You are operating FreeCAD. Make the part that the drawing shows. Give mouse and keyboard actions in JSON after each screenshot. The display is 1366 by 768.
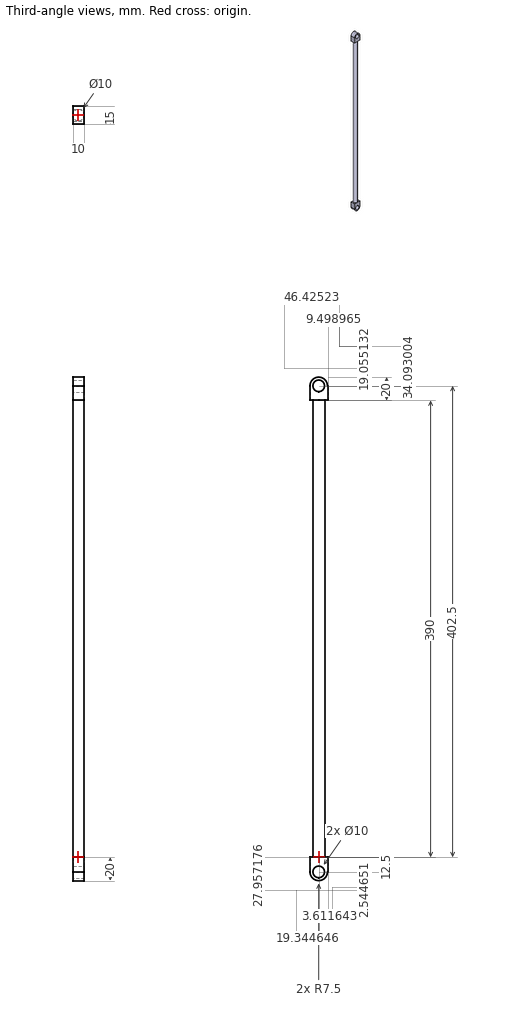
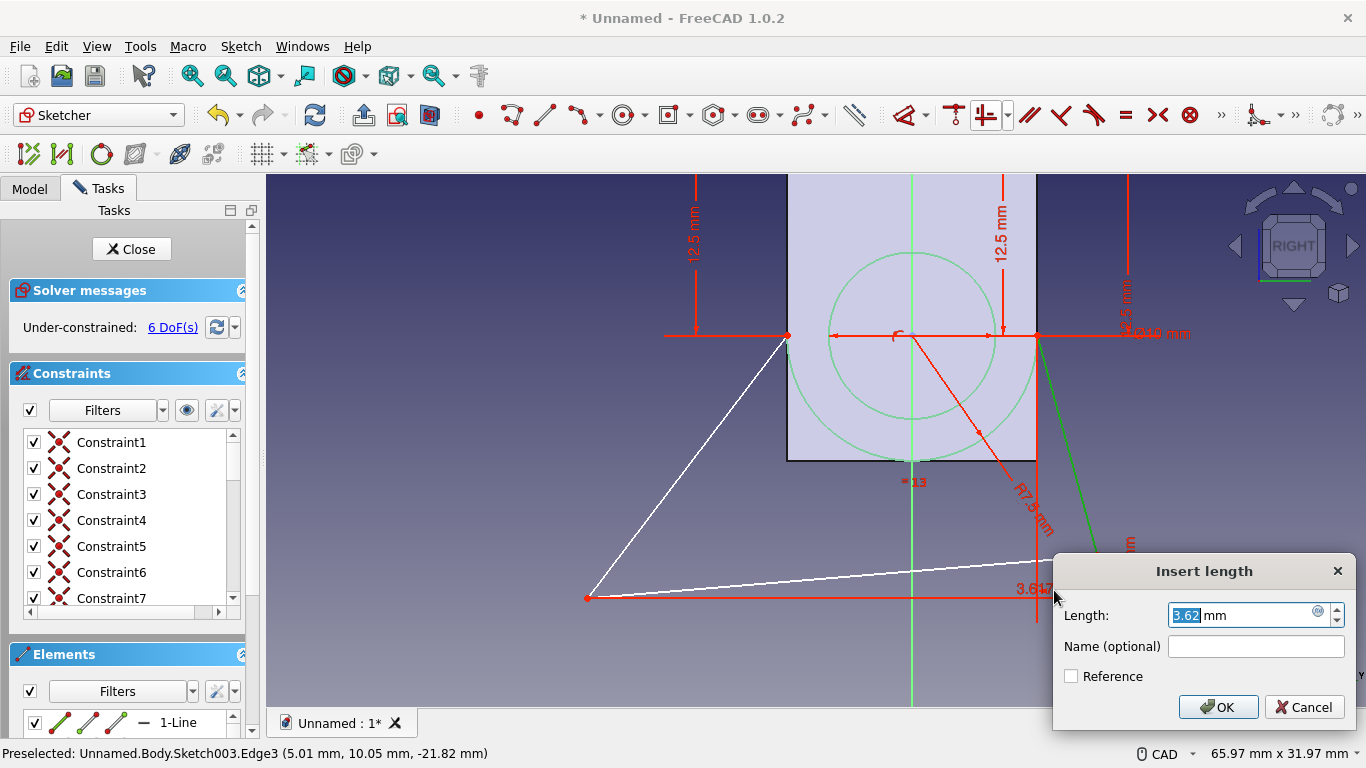
{"action": "type", "text": "3.611643"}
{"action": "key", "text": "Return"}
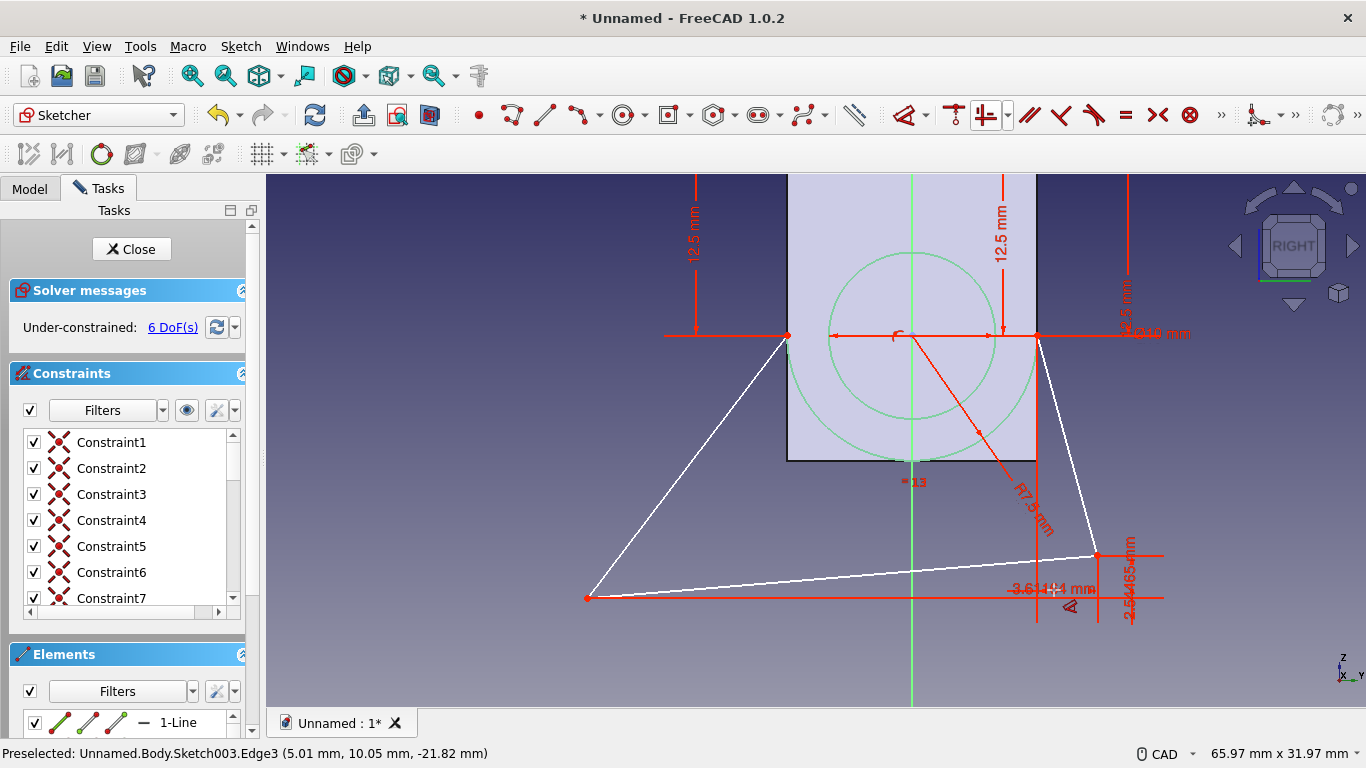
{"action": "scroll", "coordinate": [744, 635], "scroll_direction": "down", "scroll_amount": 15}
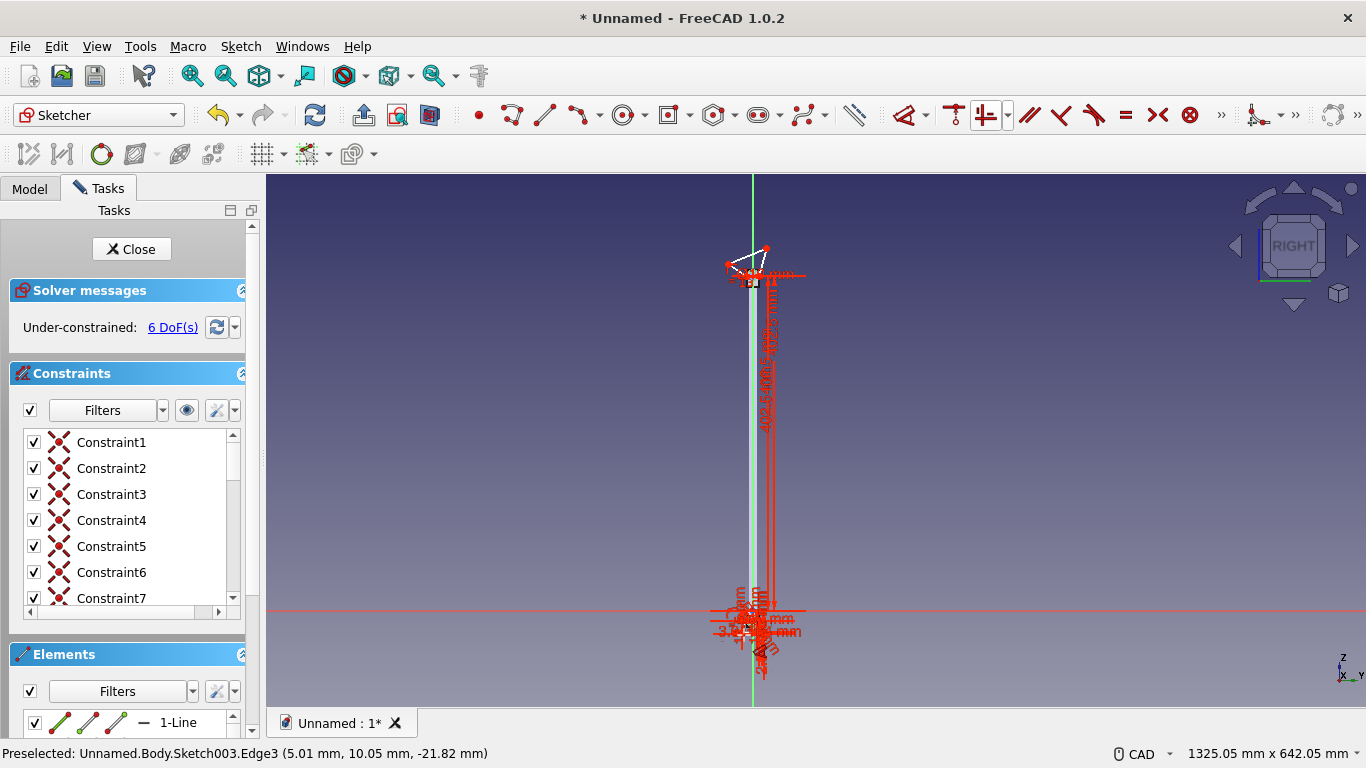
{"action": "scroll", "coordinate": [761, 268], "scroll_direction": "up", "scroll_amount": 9}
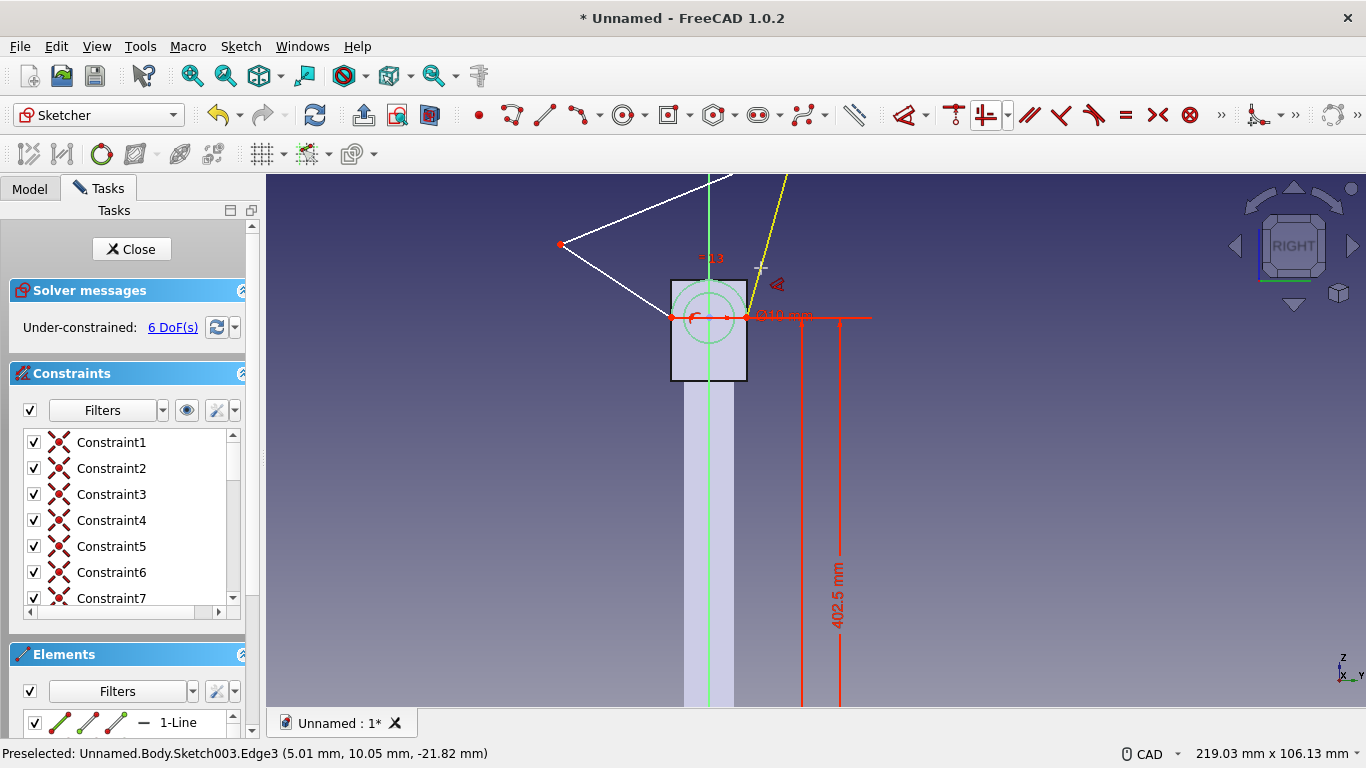
{"action": "left_click", "coordinate": [761, 267]}
{"action": "left_click", "coordinate": [770, 352]}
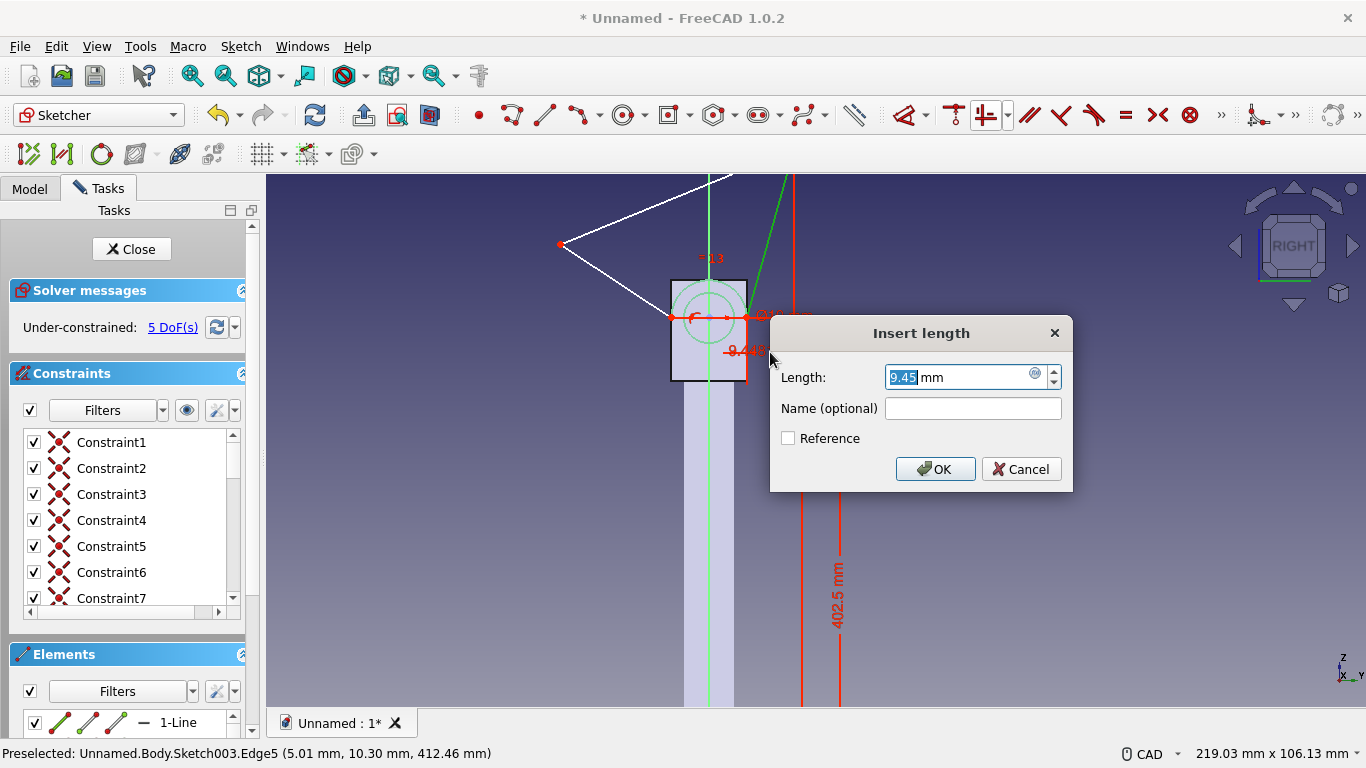
{"action": "type", "text": "9.498965"}
{"action": "key", "text": "Return"}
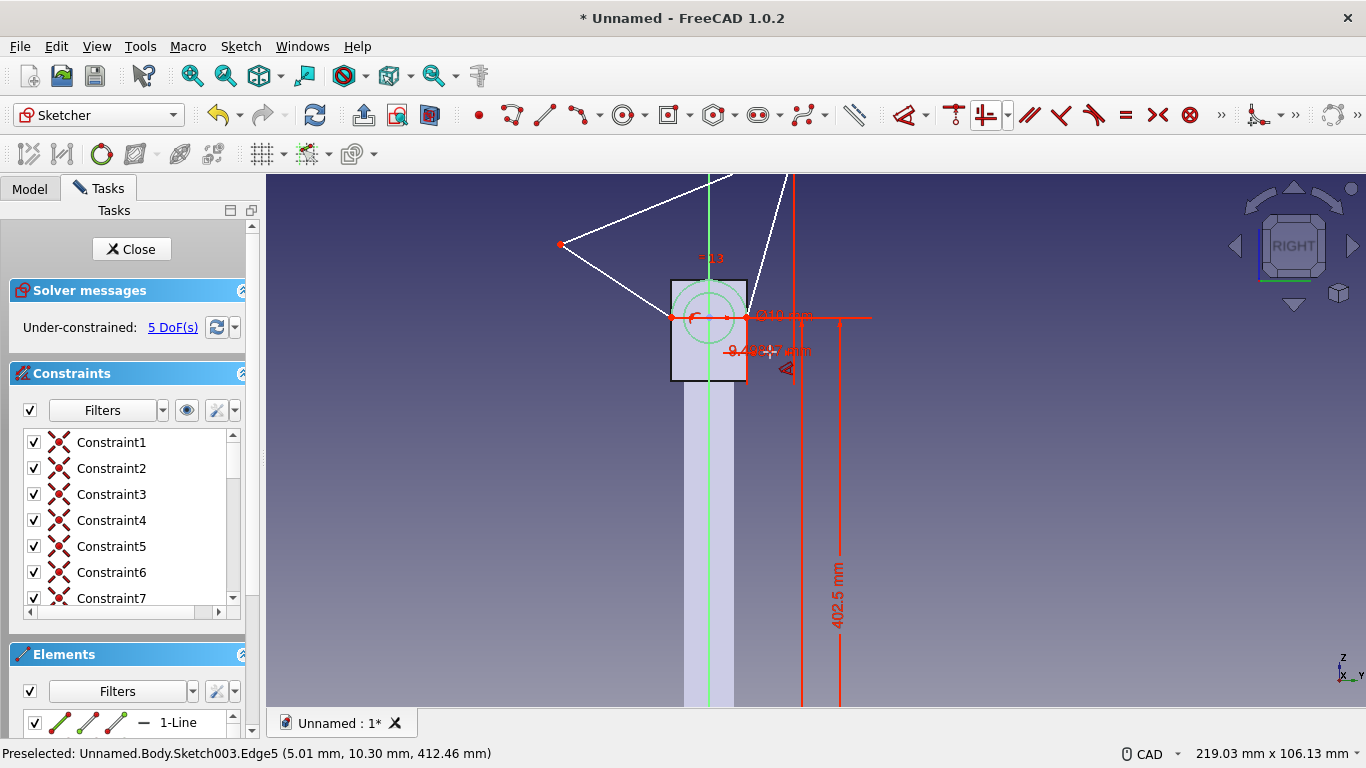
{"action": "scroll", "coordinate": [758, 304], "scroll_direction": "down", "scroll_amount": 10}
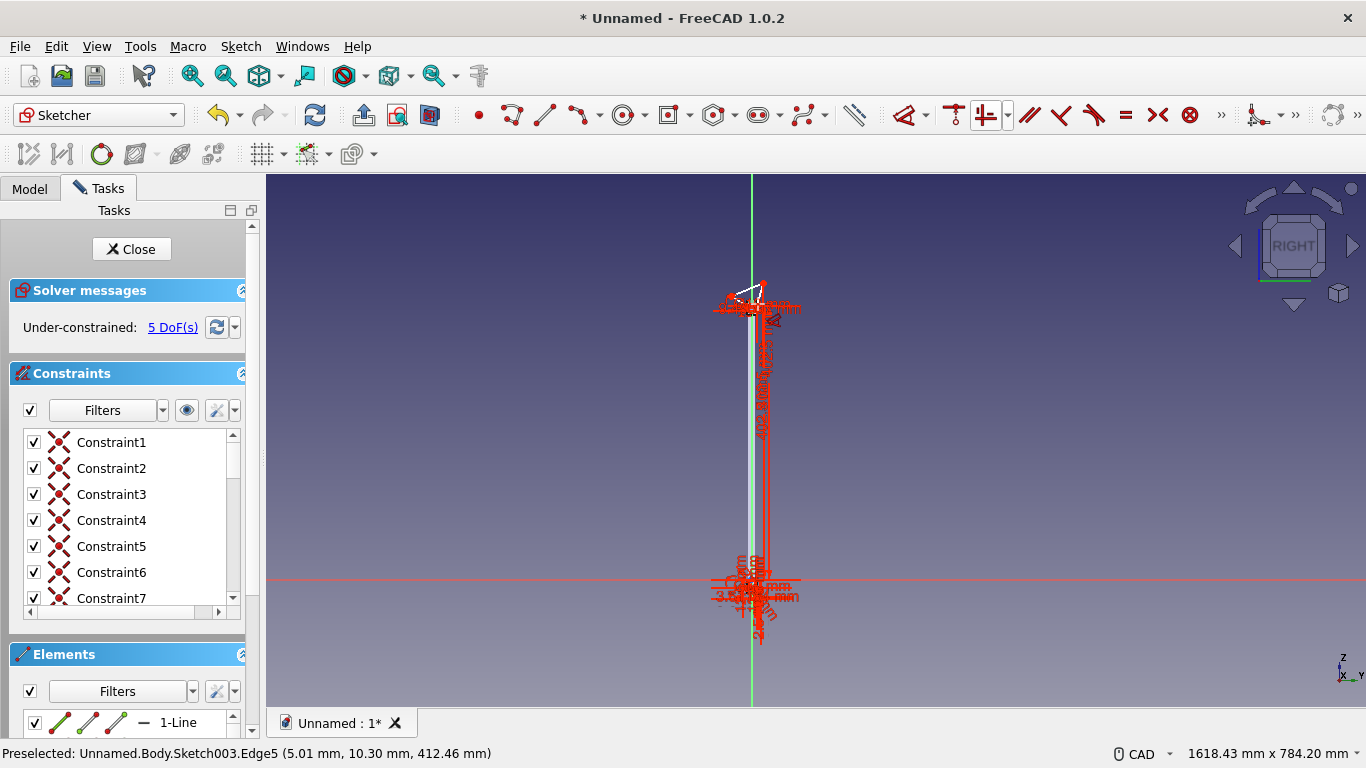
{"action": "scroll", "coordinate": [741, 292], "scroll_direction": "up", "scroll_amount": 3}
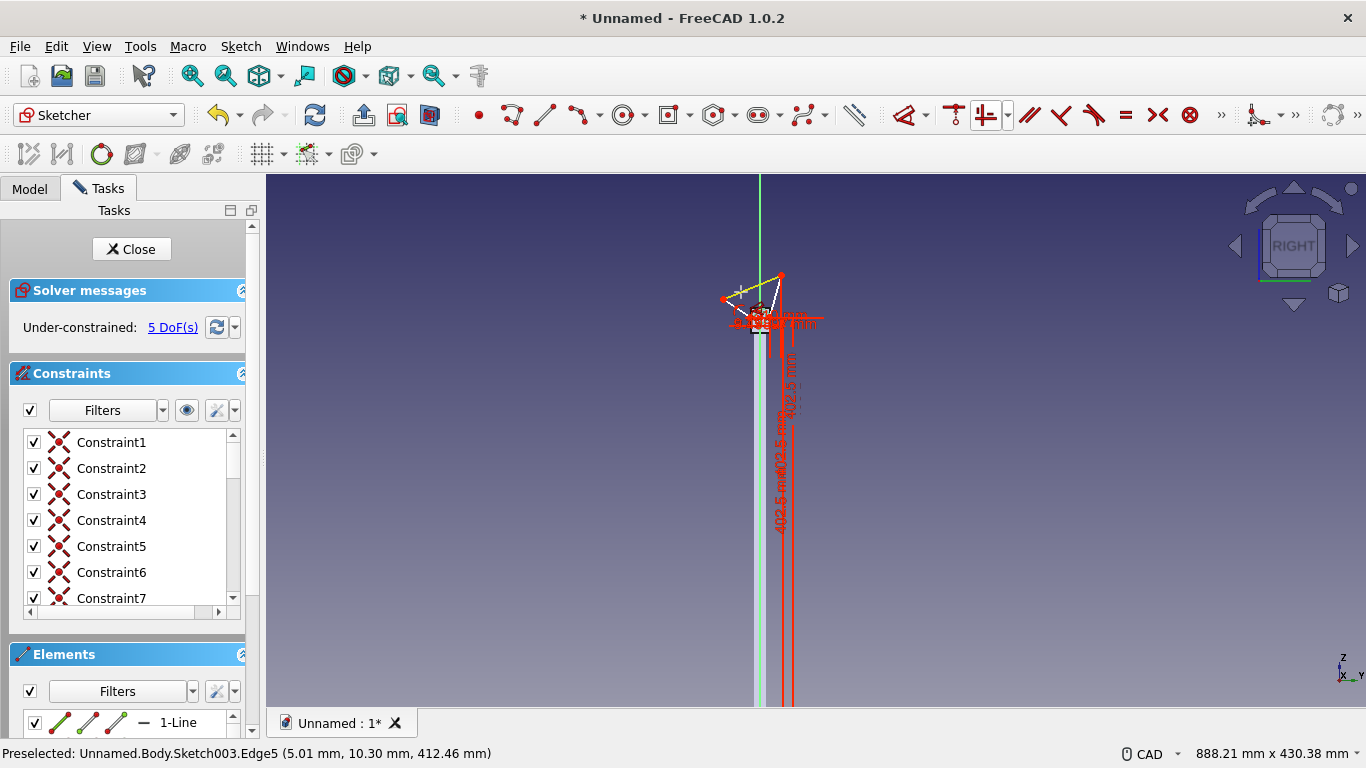
{"action": "left_click", "coordinate": [741, 292]}
{"action": "left_click", "coordinate": [739, 242]}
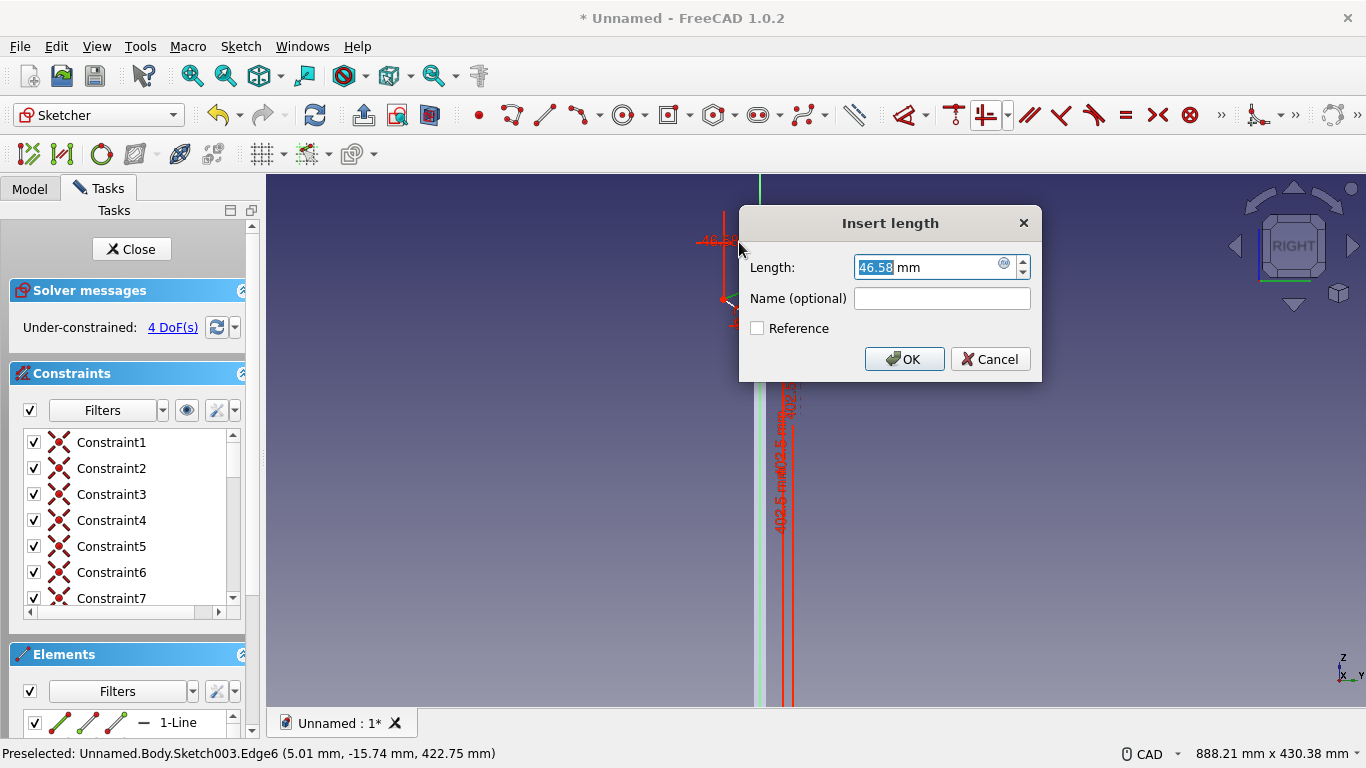
{"action": "type", "text": "46.42523"}
{"action": "key", "text": "Return"}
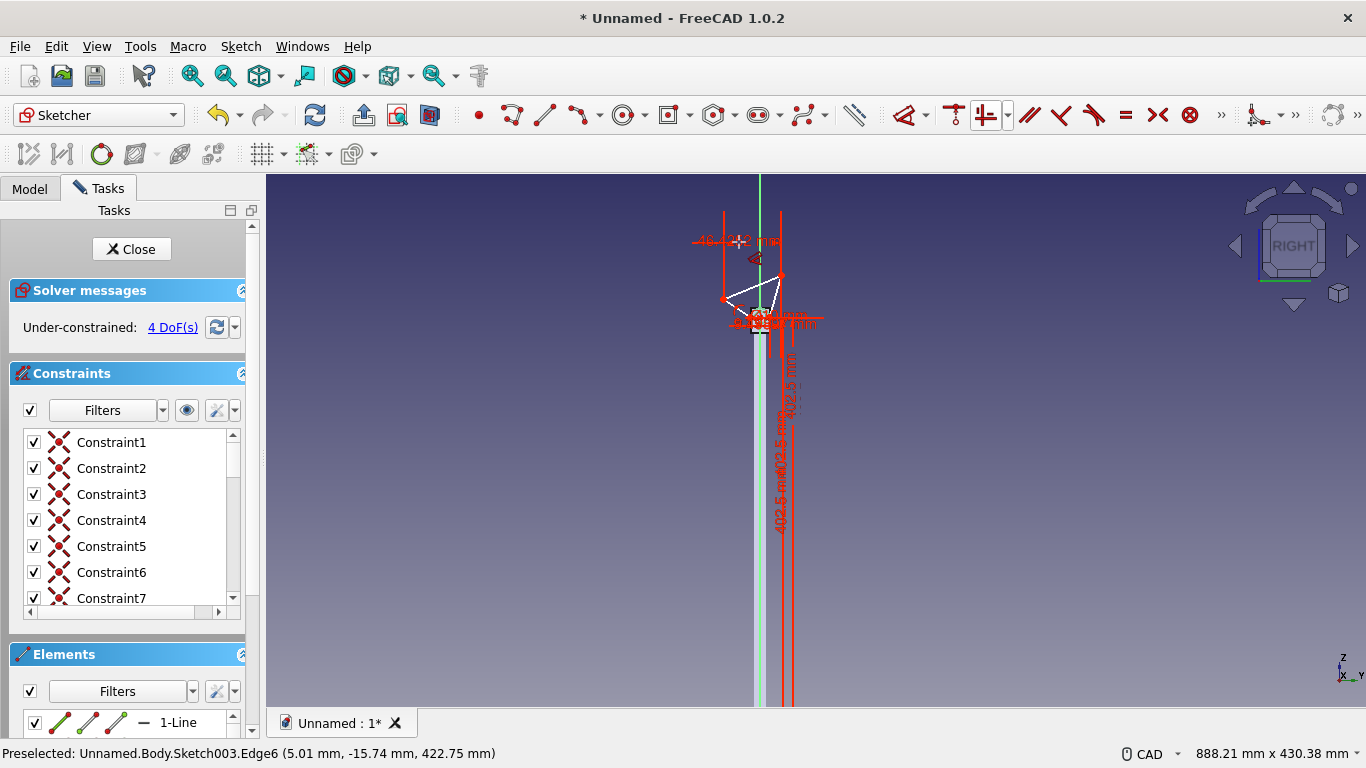
{"action": "scroll", "coordinate": [741, 292], "scroll_direction": "down", "scroll_amount": 3}